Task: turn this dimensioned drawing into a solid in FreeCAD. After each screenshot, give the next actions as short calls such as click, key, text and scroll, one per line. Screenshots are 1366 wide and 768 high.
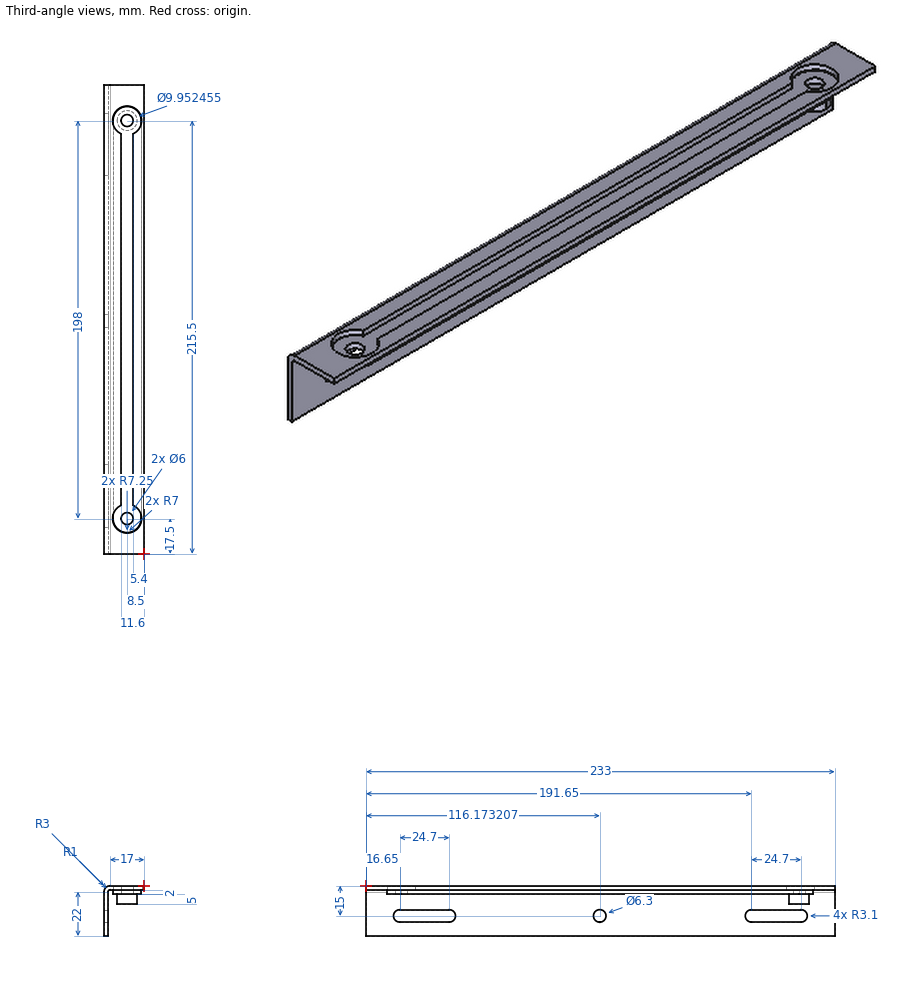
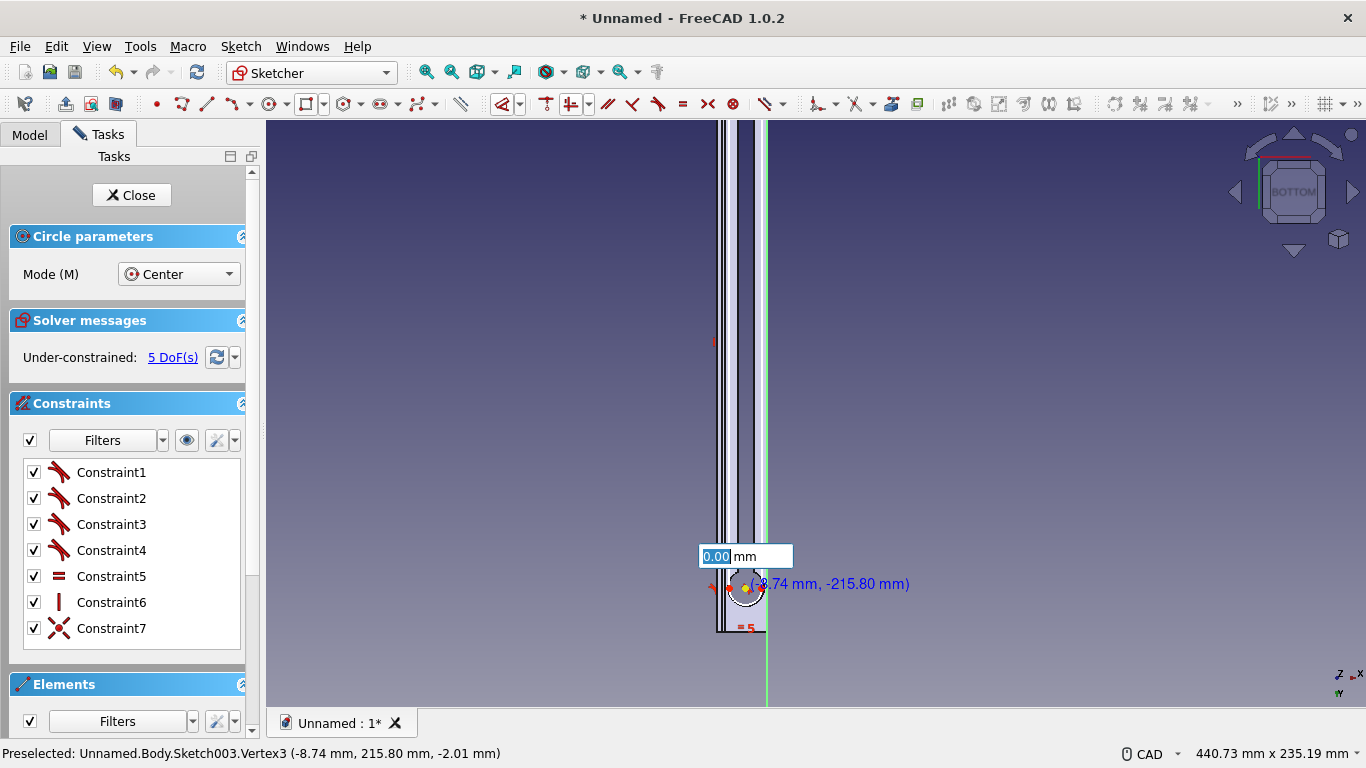
scroll(753, 585, up, 4)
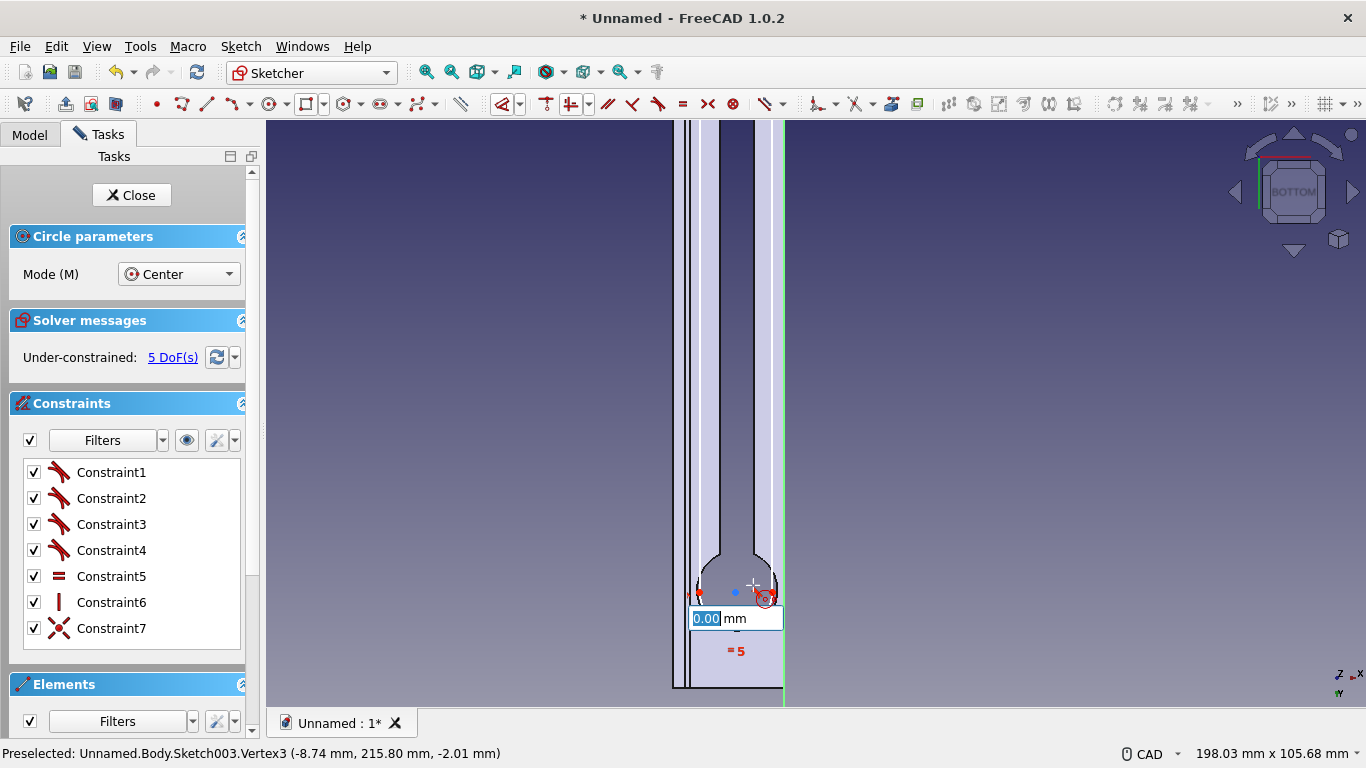
click(753, 585)
key(Escape)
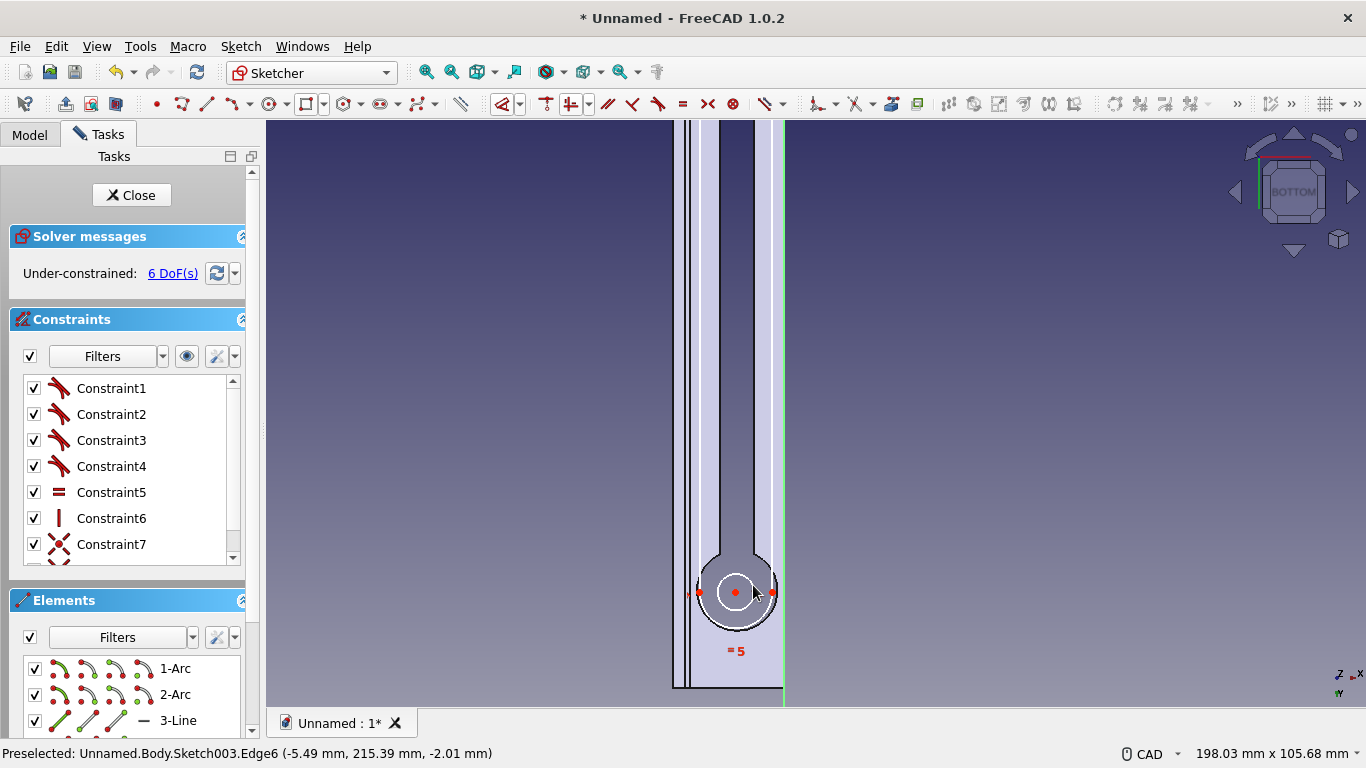
scroll(750, 587, down, 6)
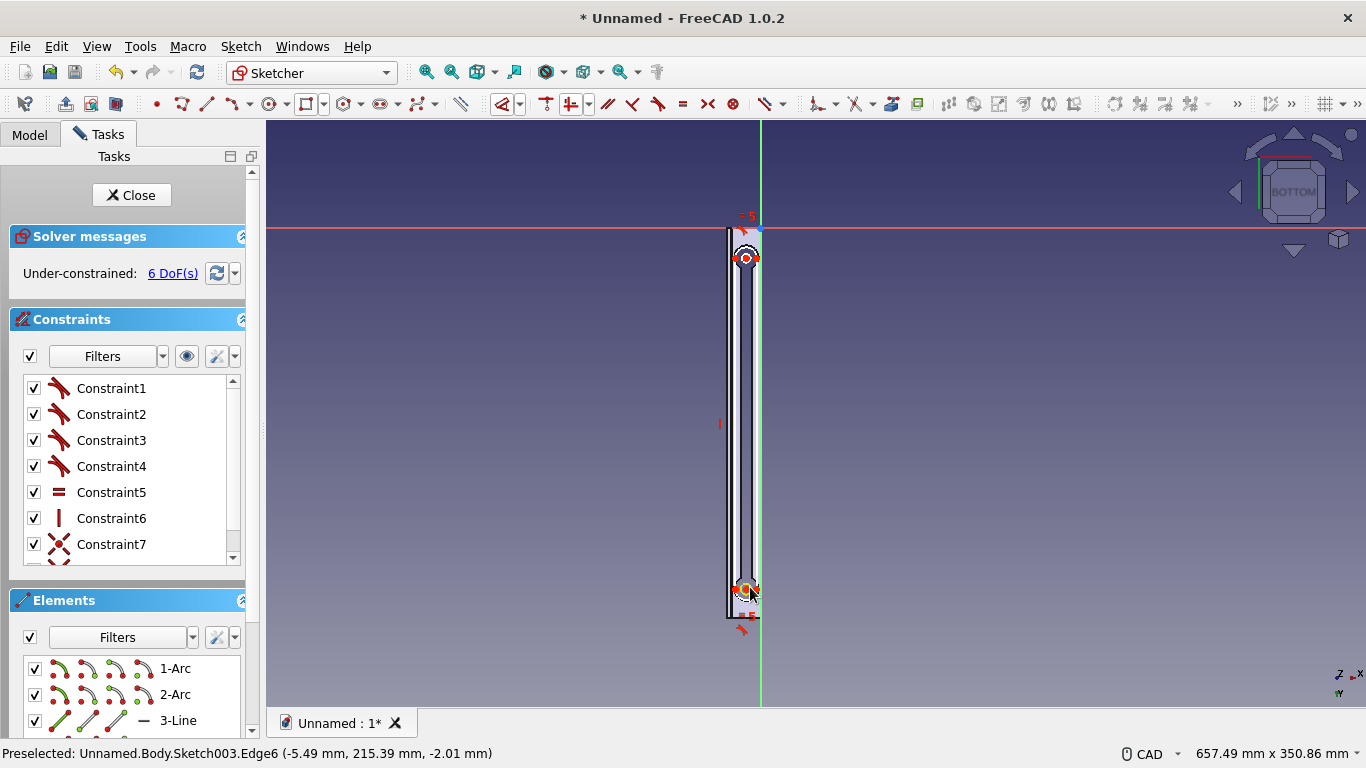
scroll(749, 255, up, 6)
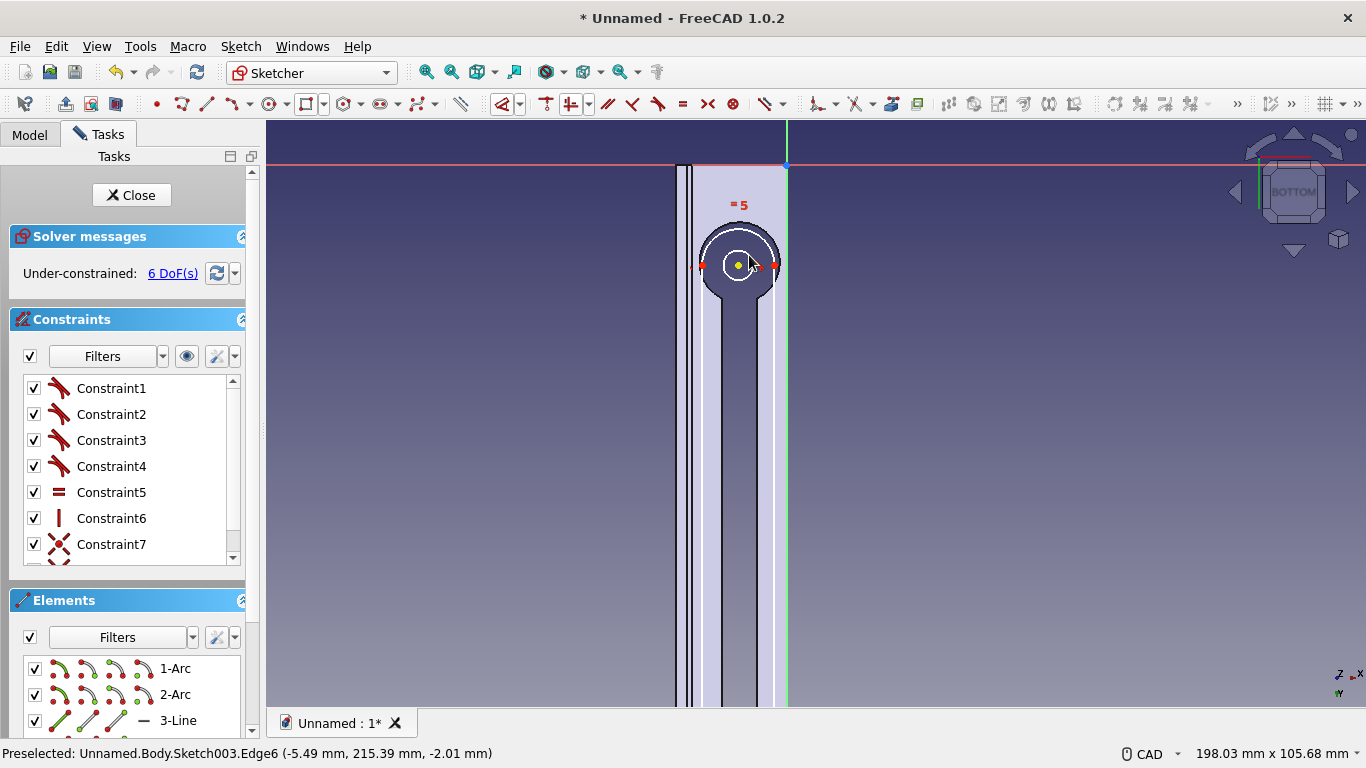
click(749, 255)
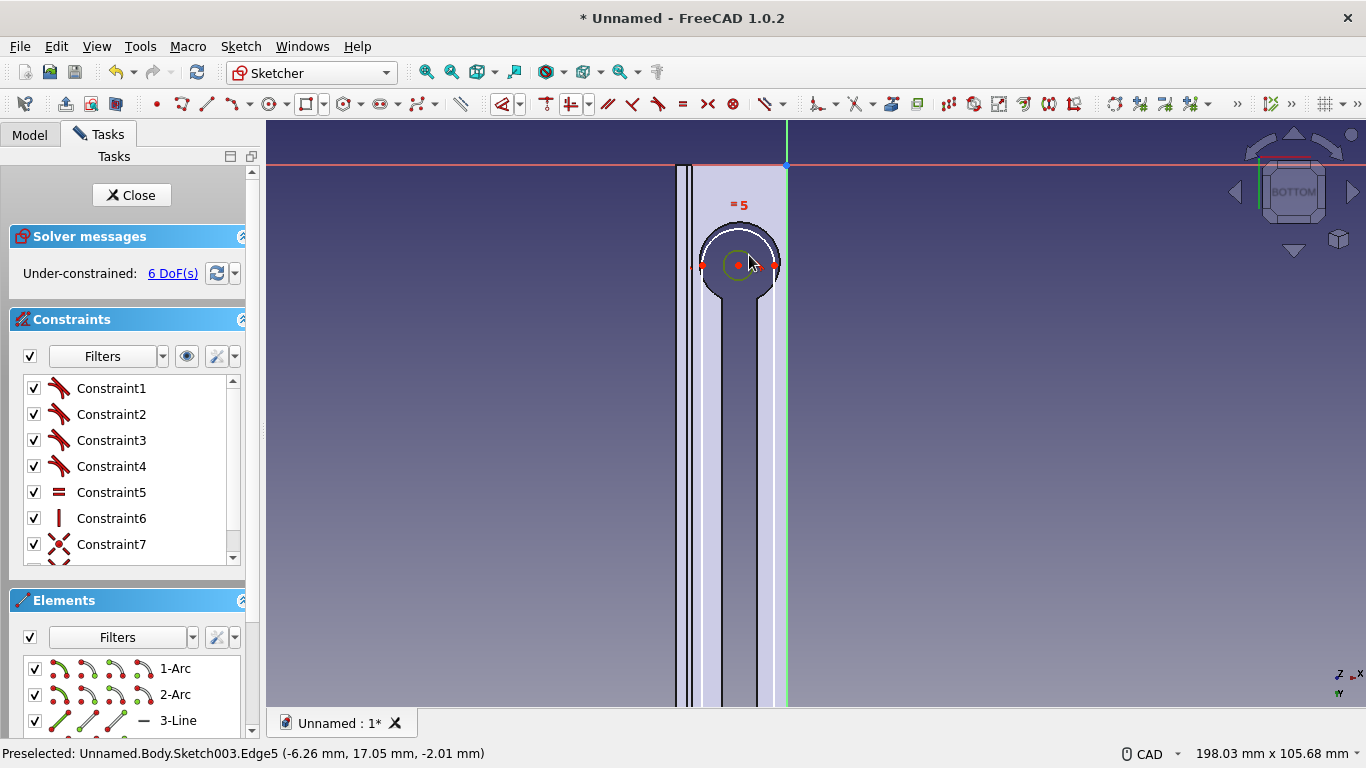
scroll(749, 254, down, 6)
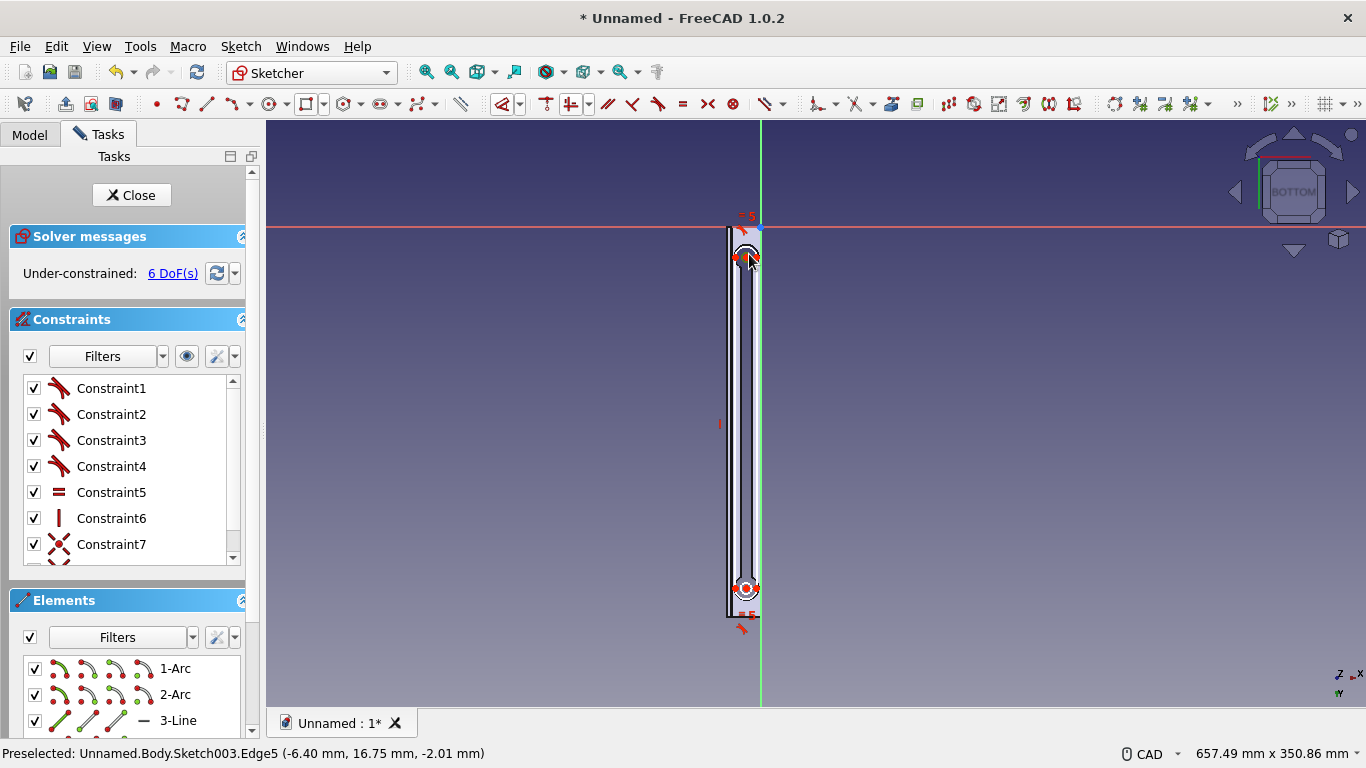
scroll(750, 585, up, 5)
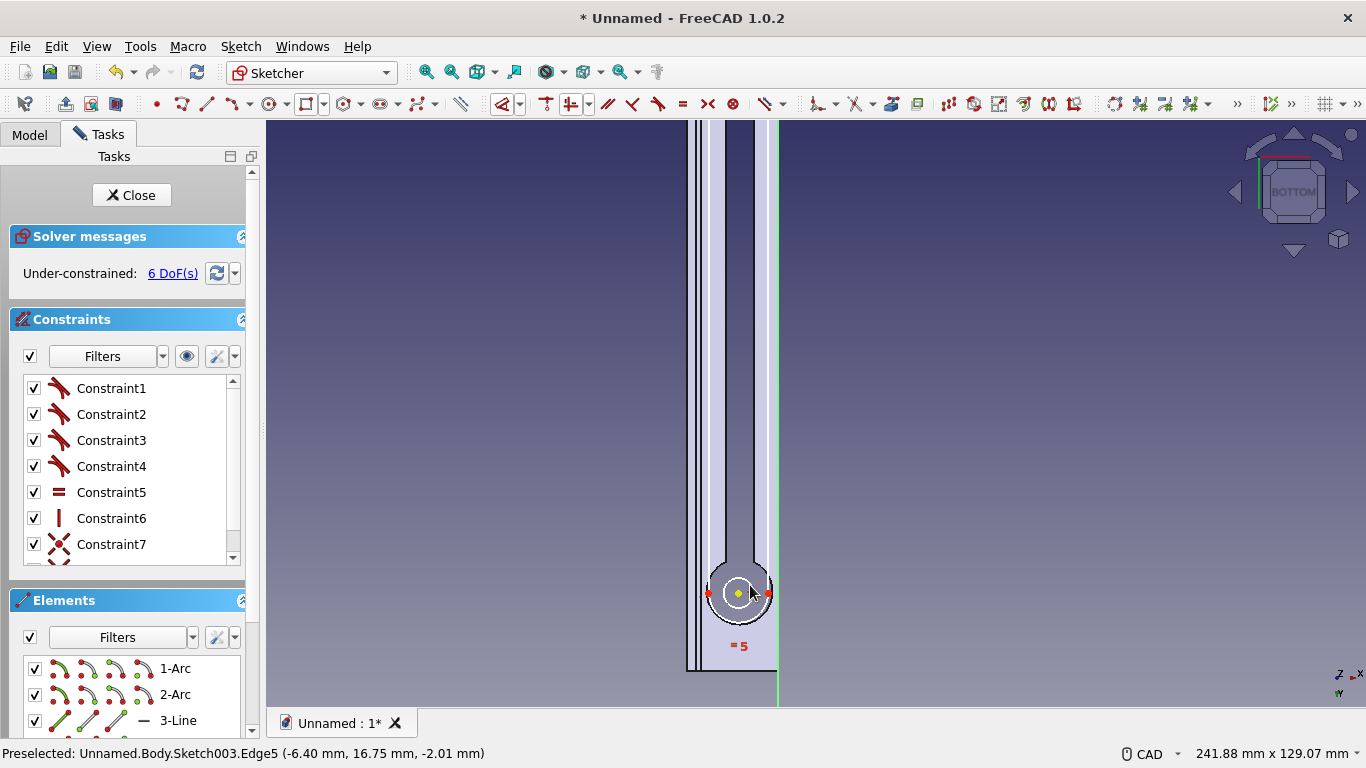
click(749, 582)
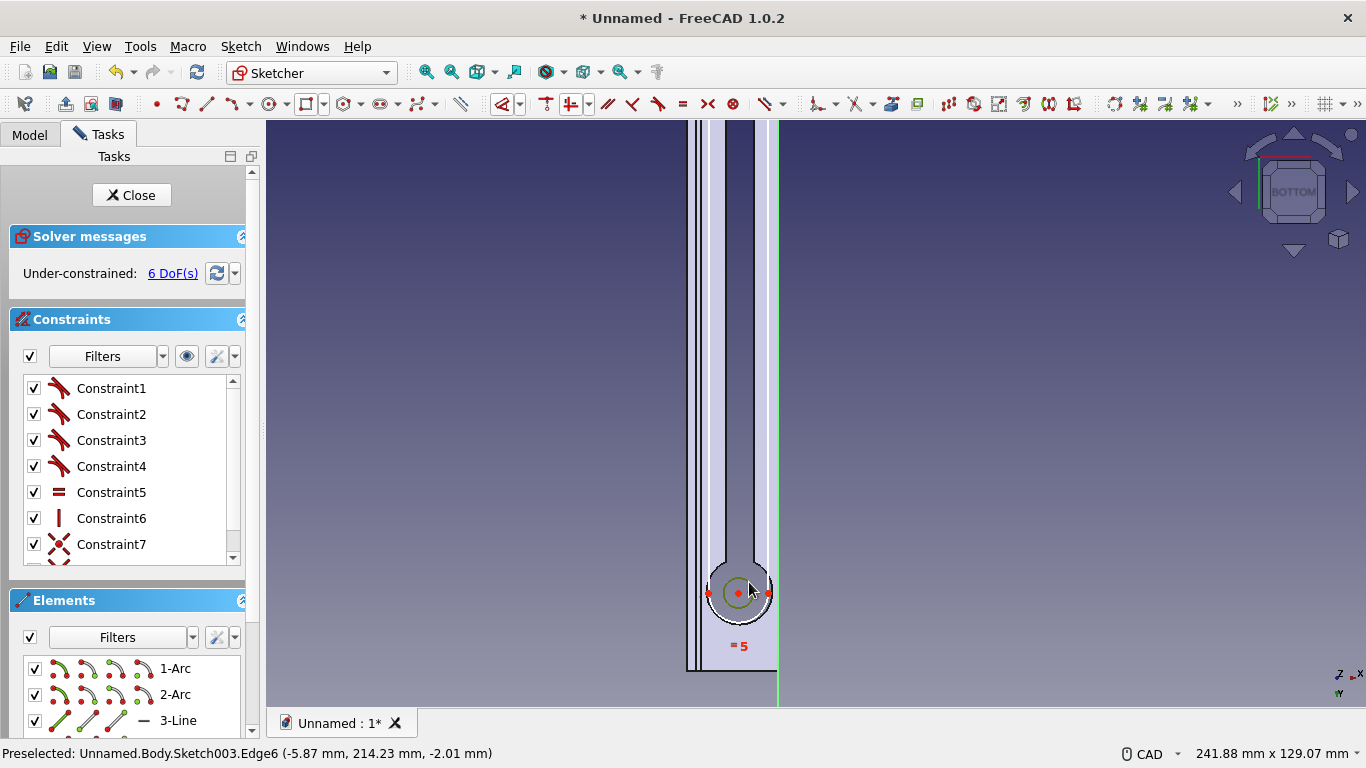
click(683, 104)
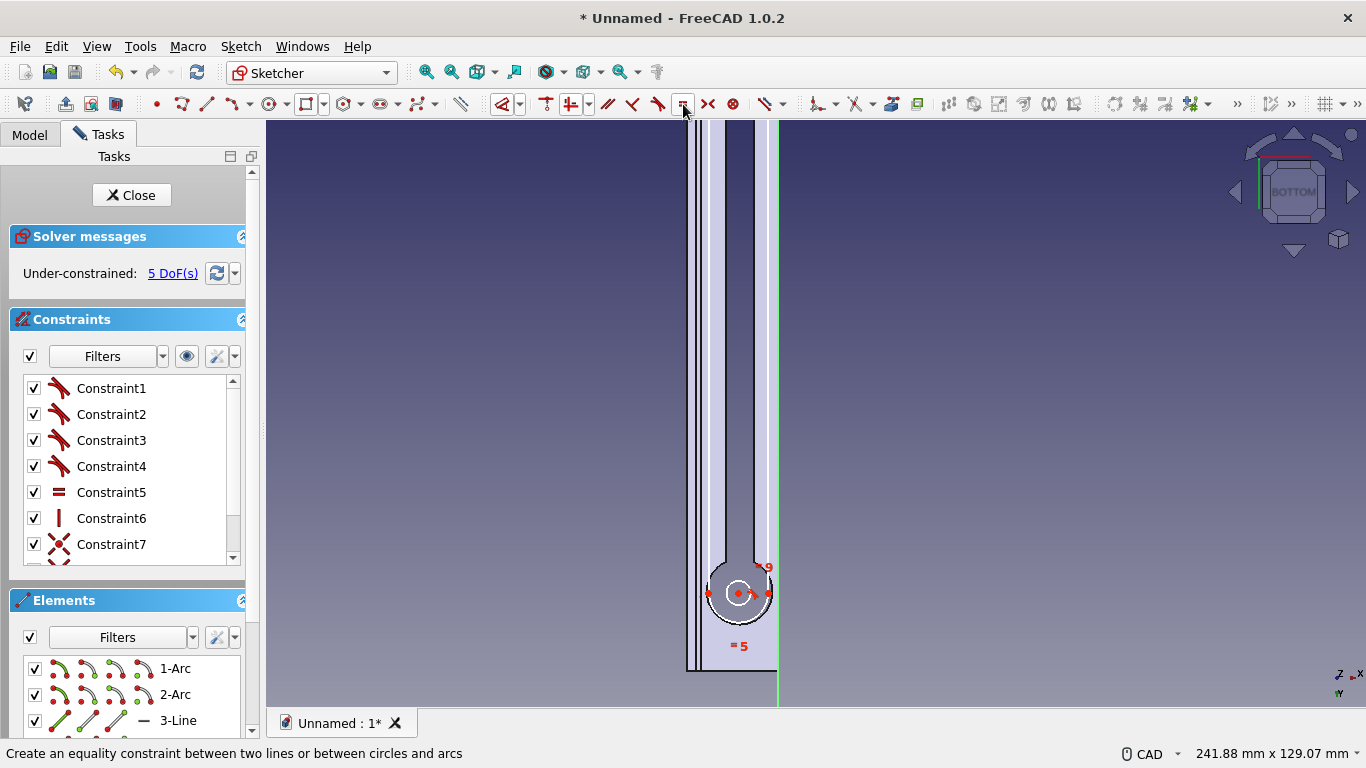
scroll(721, 617, up, 2)